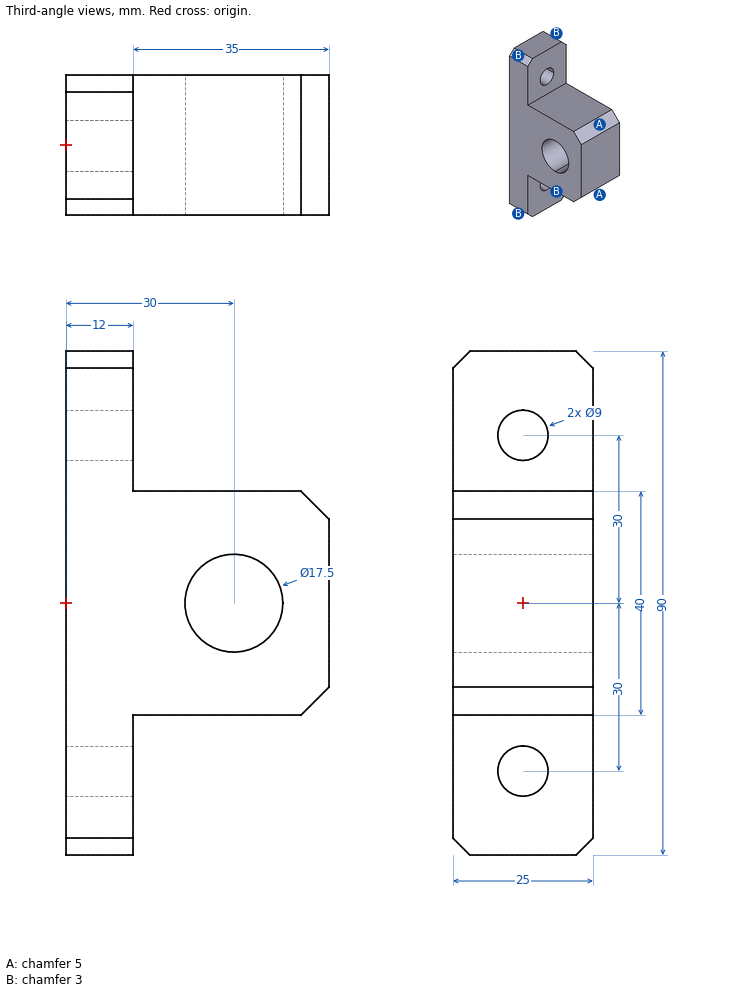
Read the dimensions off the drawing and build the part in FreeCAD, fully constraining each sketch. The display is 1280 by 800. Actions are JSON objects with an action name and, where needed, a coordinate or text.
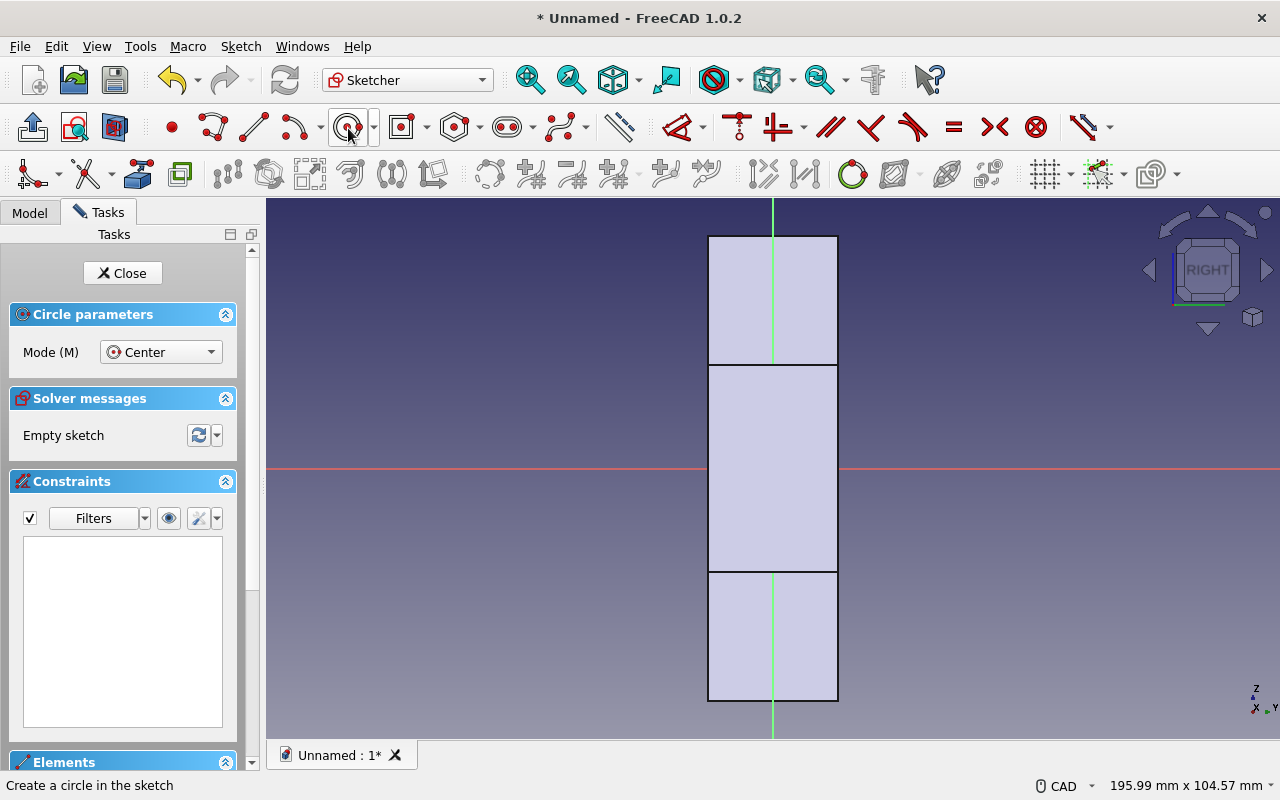
{"action": "left_click", "coordinate": [773, 313]}
{"action": "left_click", "coordinate": [789, 297]}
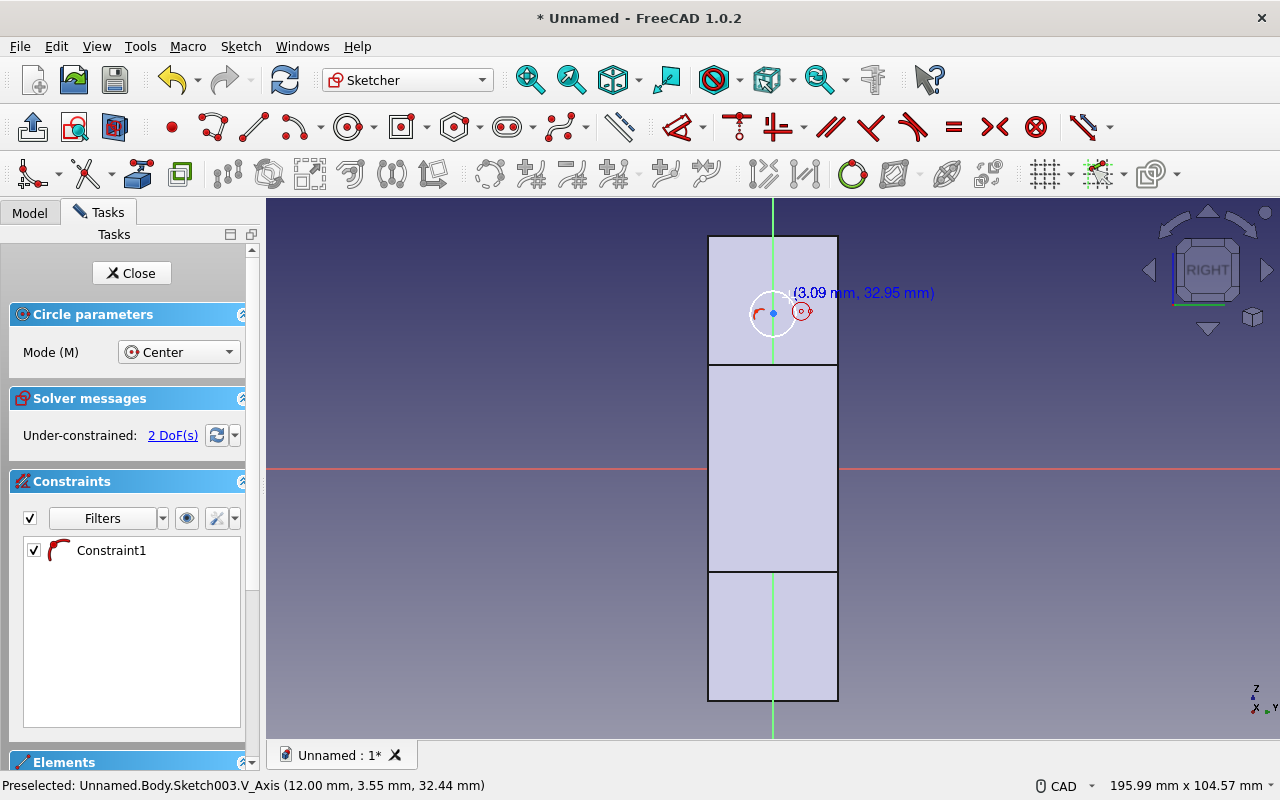
{"action": "left_click", "coordinate": [773, 624]}
{"action": "left_click", "coordinate": [789, 607]}
{"action": "key", "text": "Escape"}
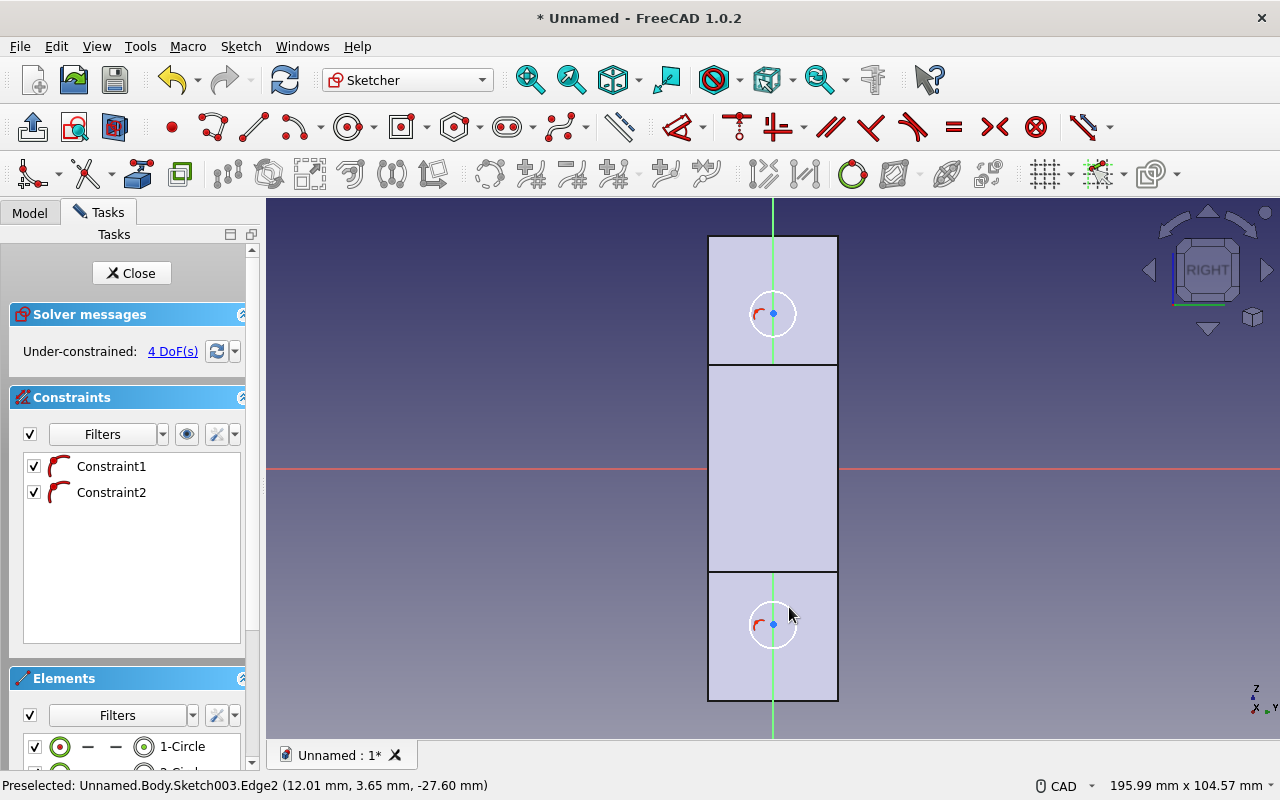
{"action": "left_click", "coordinate": [789, 298]}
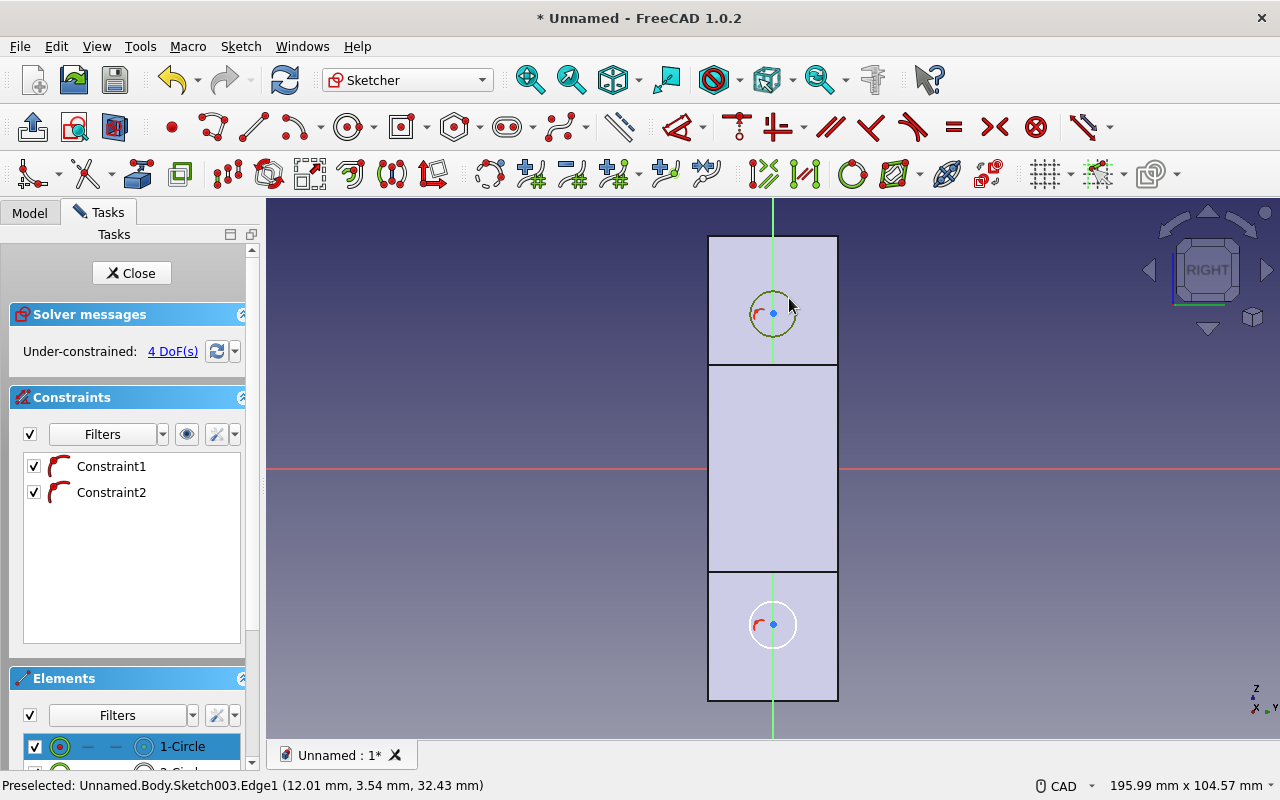
{"action": "left_click", "coordinate": [789, 608]}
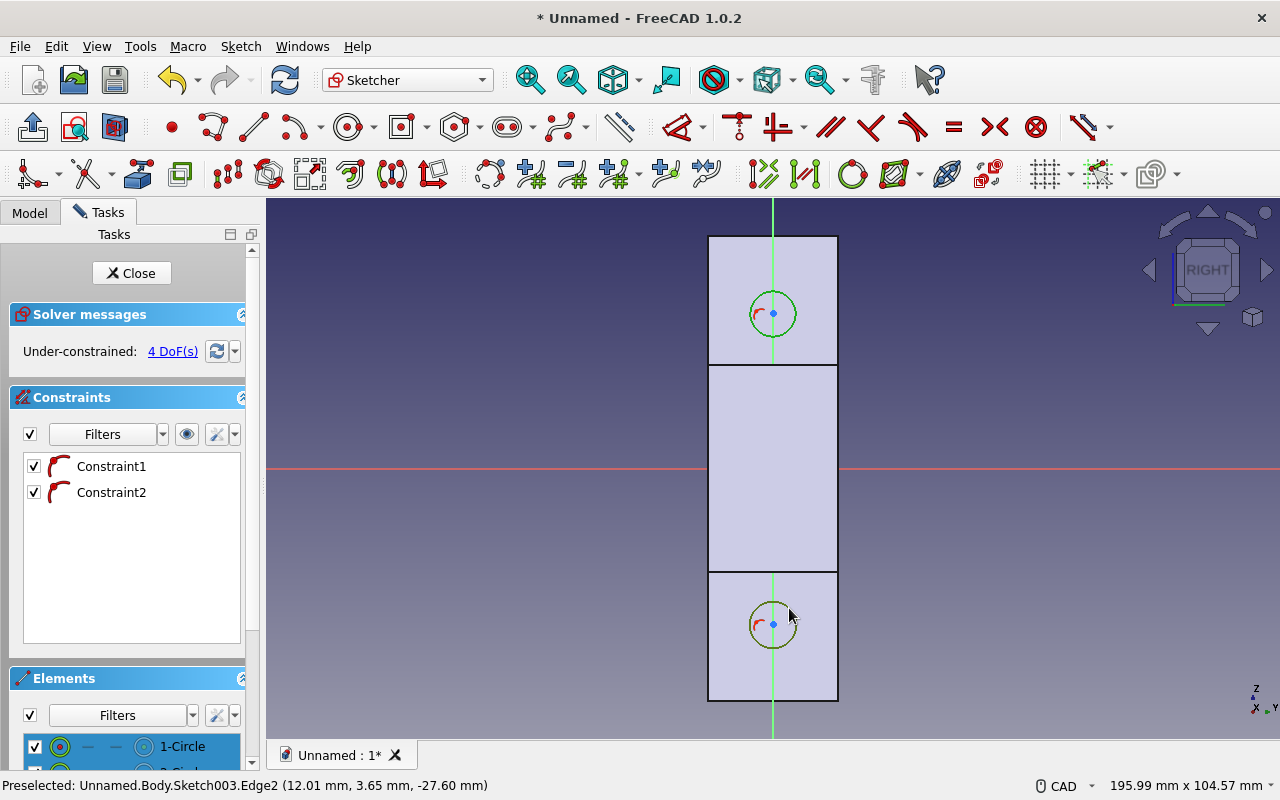
{"action": "left_click", "coordinate": [954, 128]}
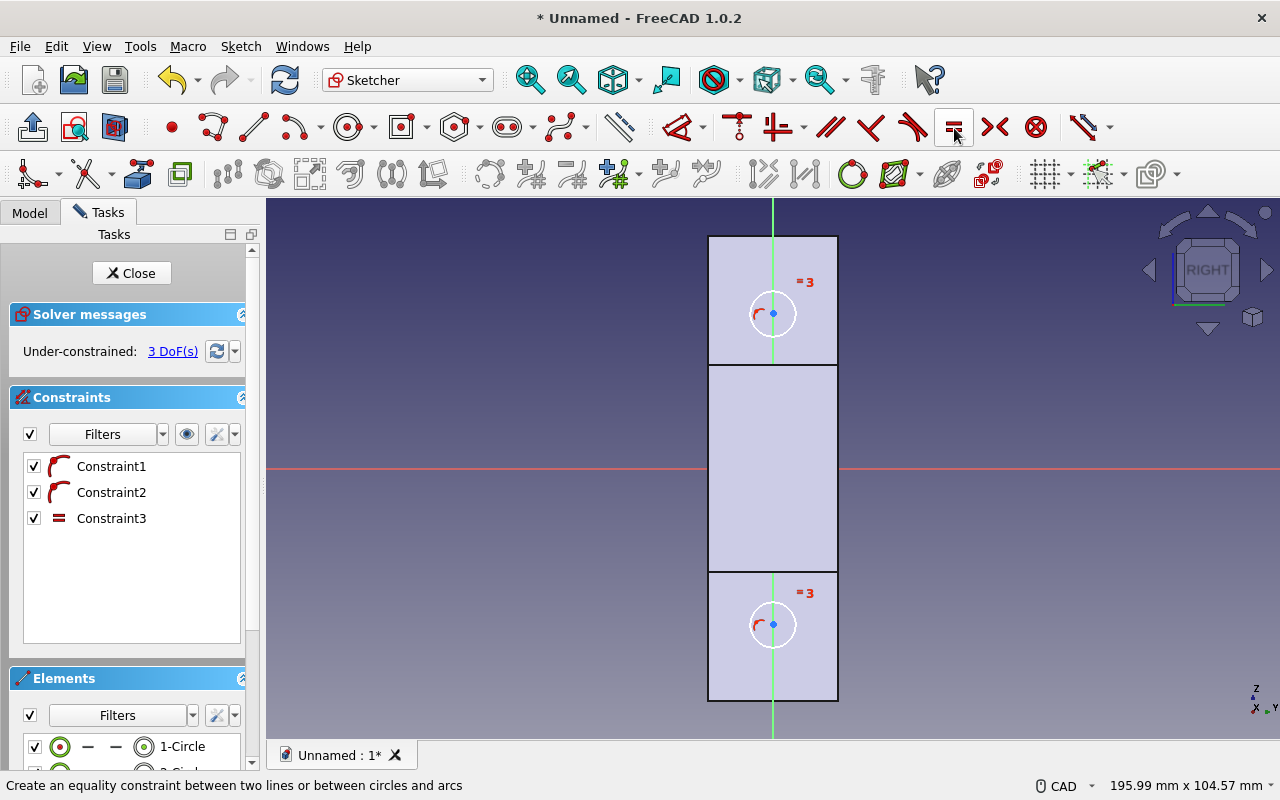
{"action": "left_click", "coordinate": [676, 128]}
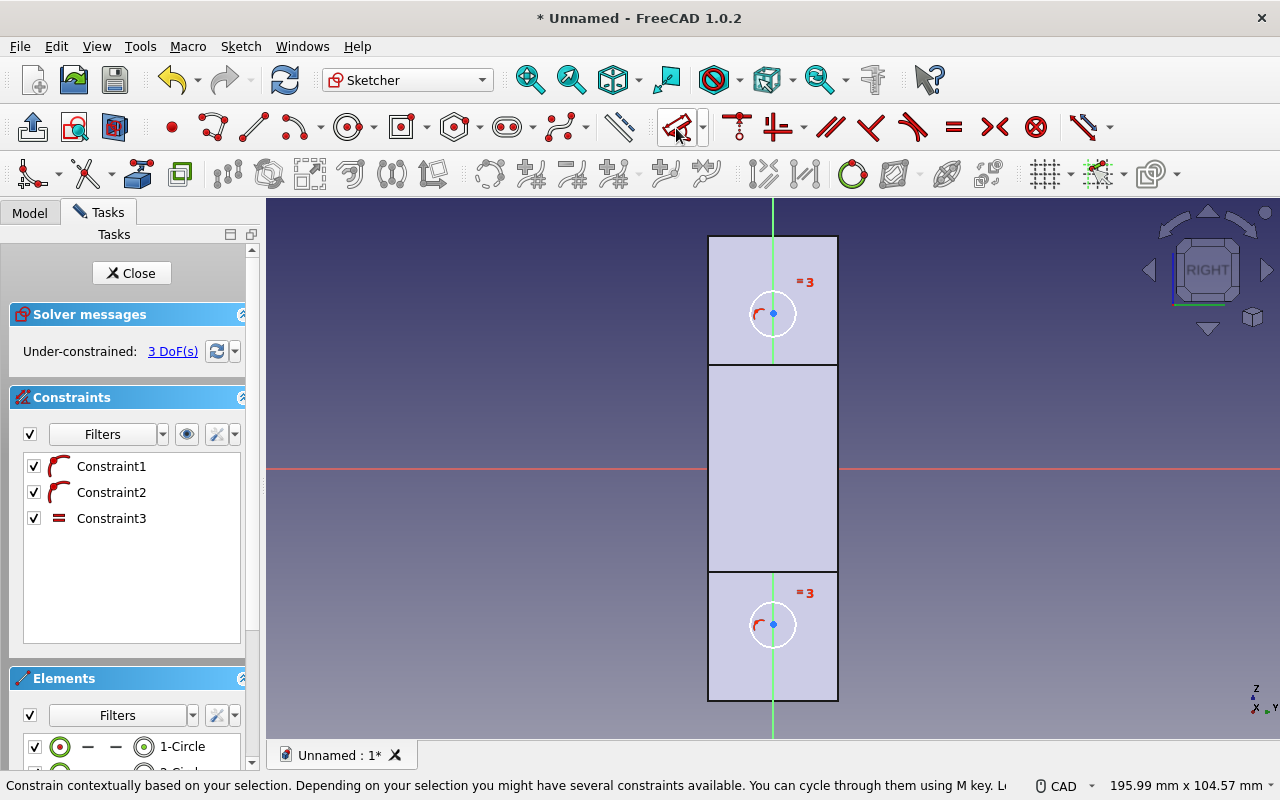
{"action": "left_click", "coordinate": [789, 298]}
{"action": "left_click", "coordinate": [812, 275]}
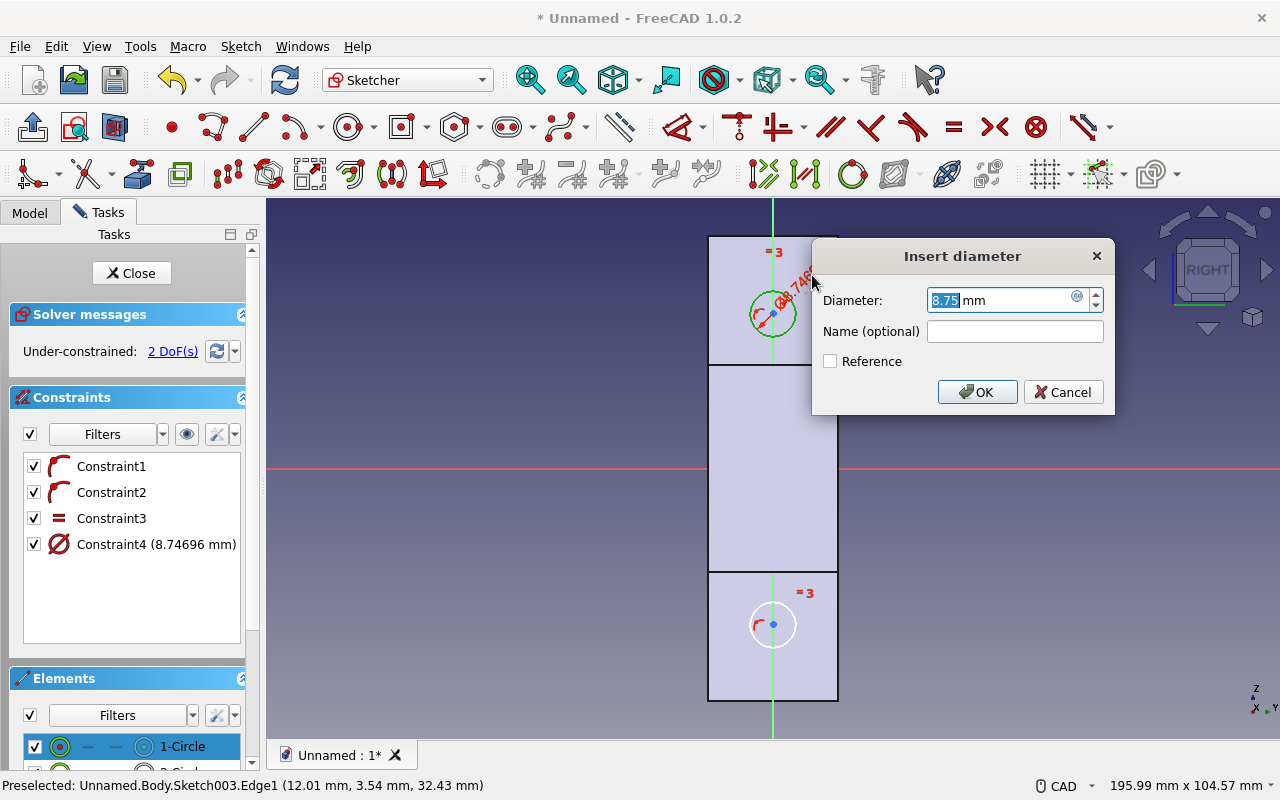
{"action": "type", "text": "9"}
{"action": "key", "text": "Return"}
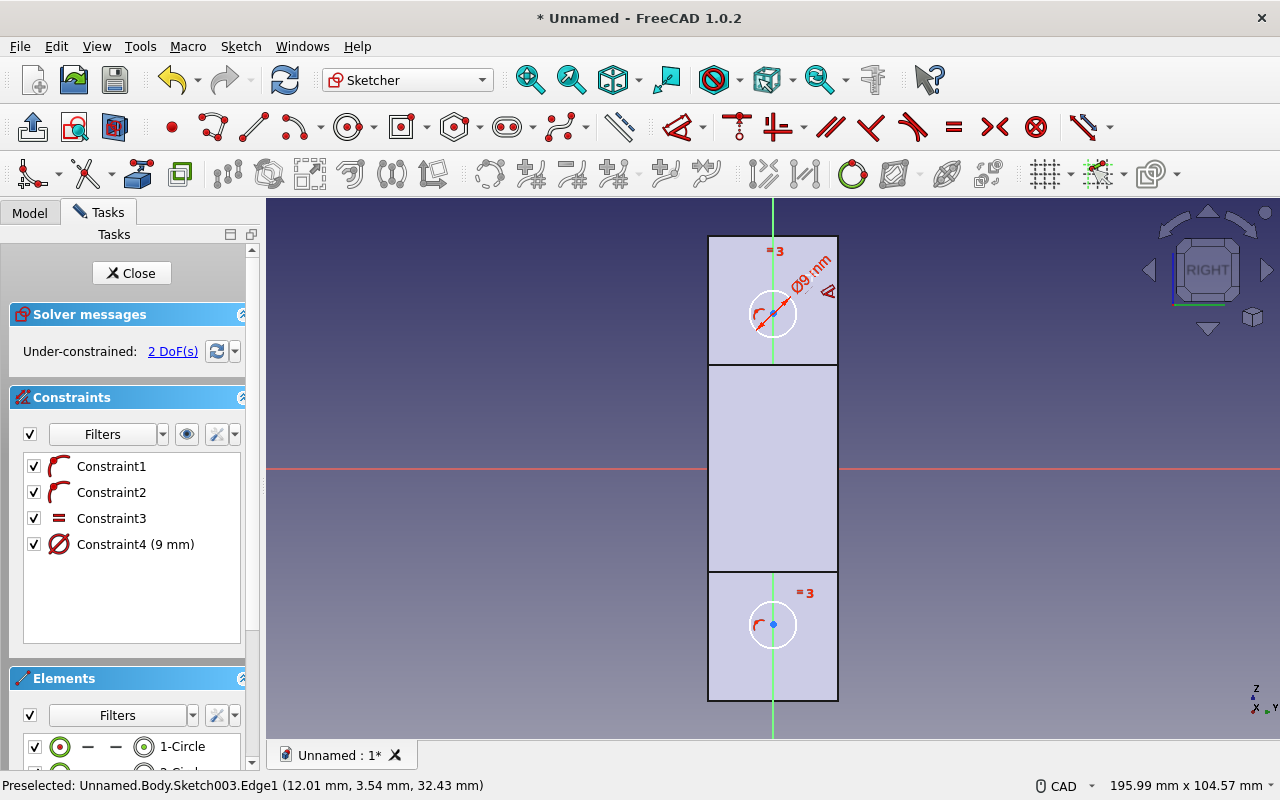
{"action": "left_click", "coordinate": [773, 314]}
{"action": "left_click", "coordinate": [807, 391]}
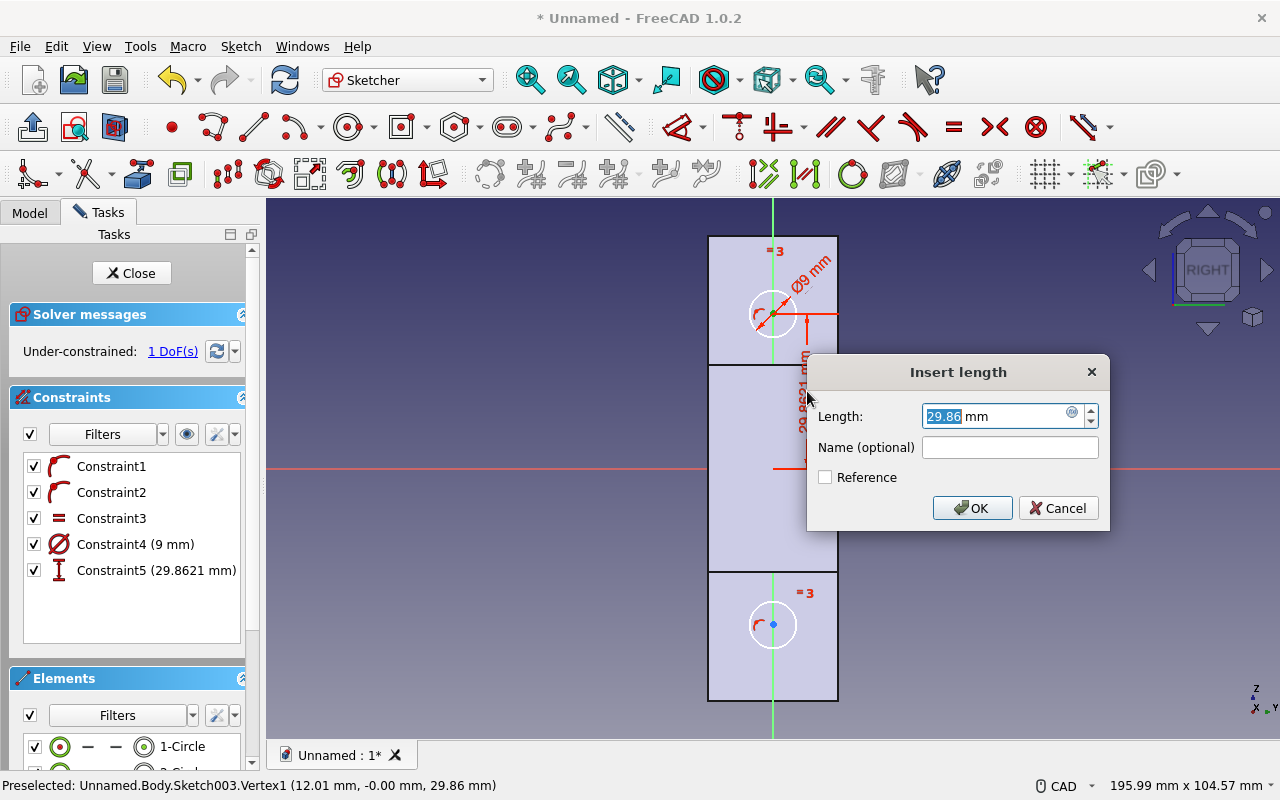
{"action": "type", "text": "30"}
{"action": "key", "text": "Return"}